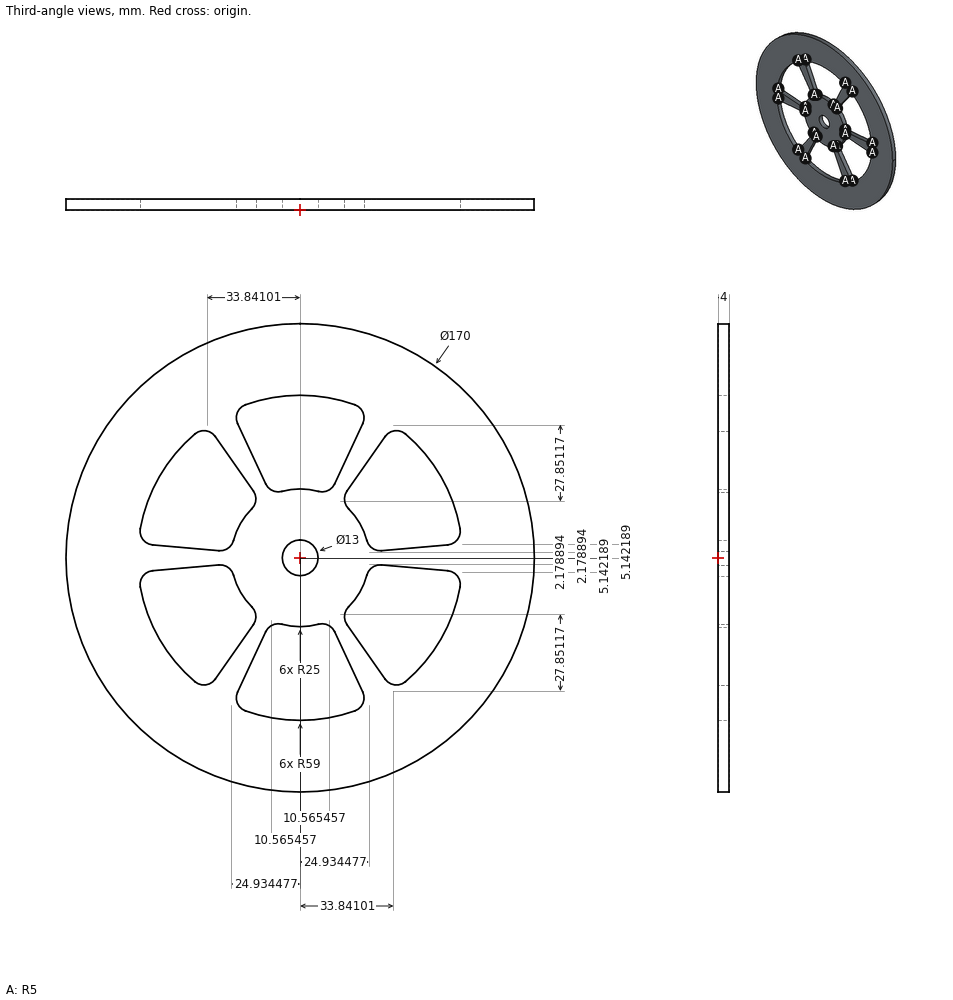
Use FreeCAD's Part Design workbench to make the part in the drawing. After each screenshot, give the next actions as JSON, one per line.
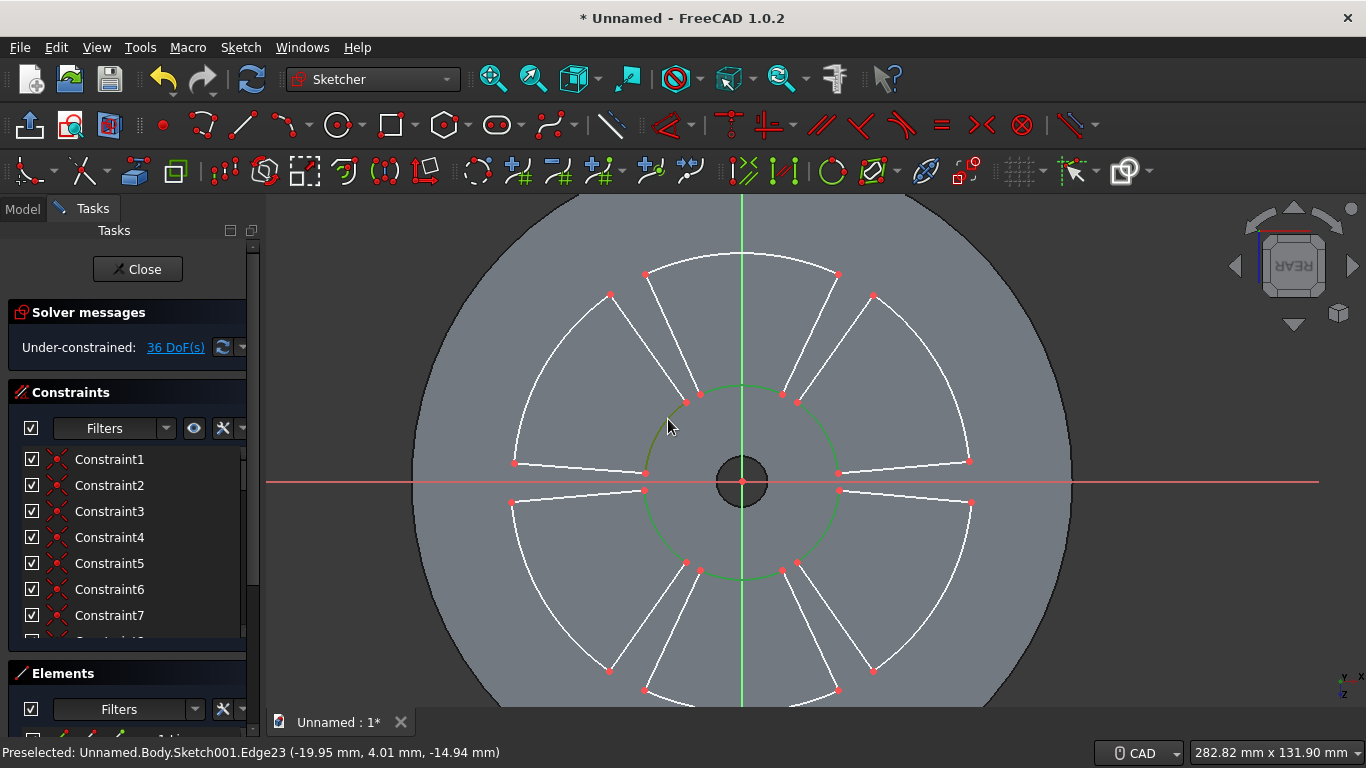
{"action": "left_click", "coordinate": [942, 126]}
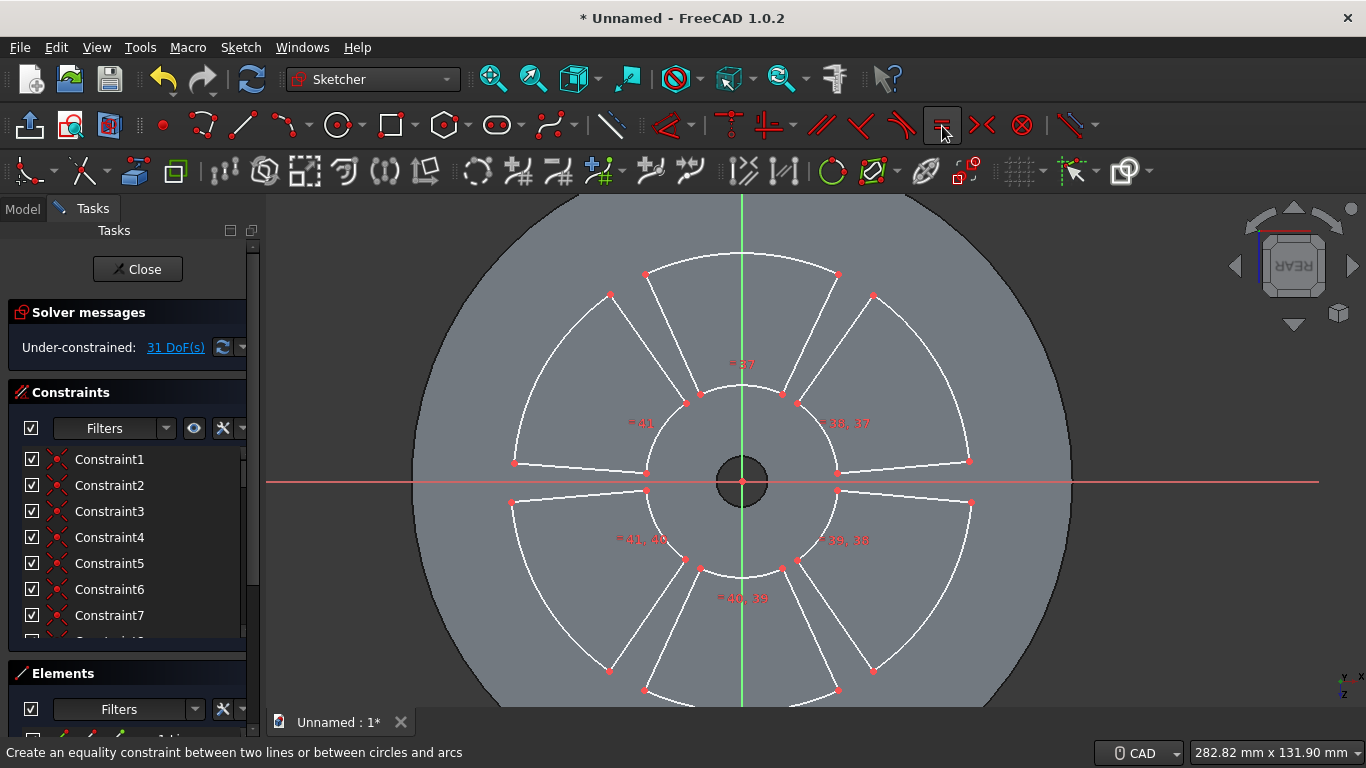
{"action": "left_click", "coordinate": [782, 257]}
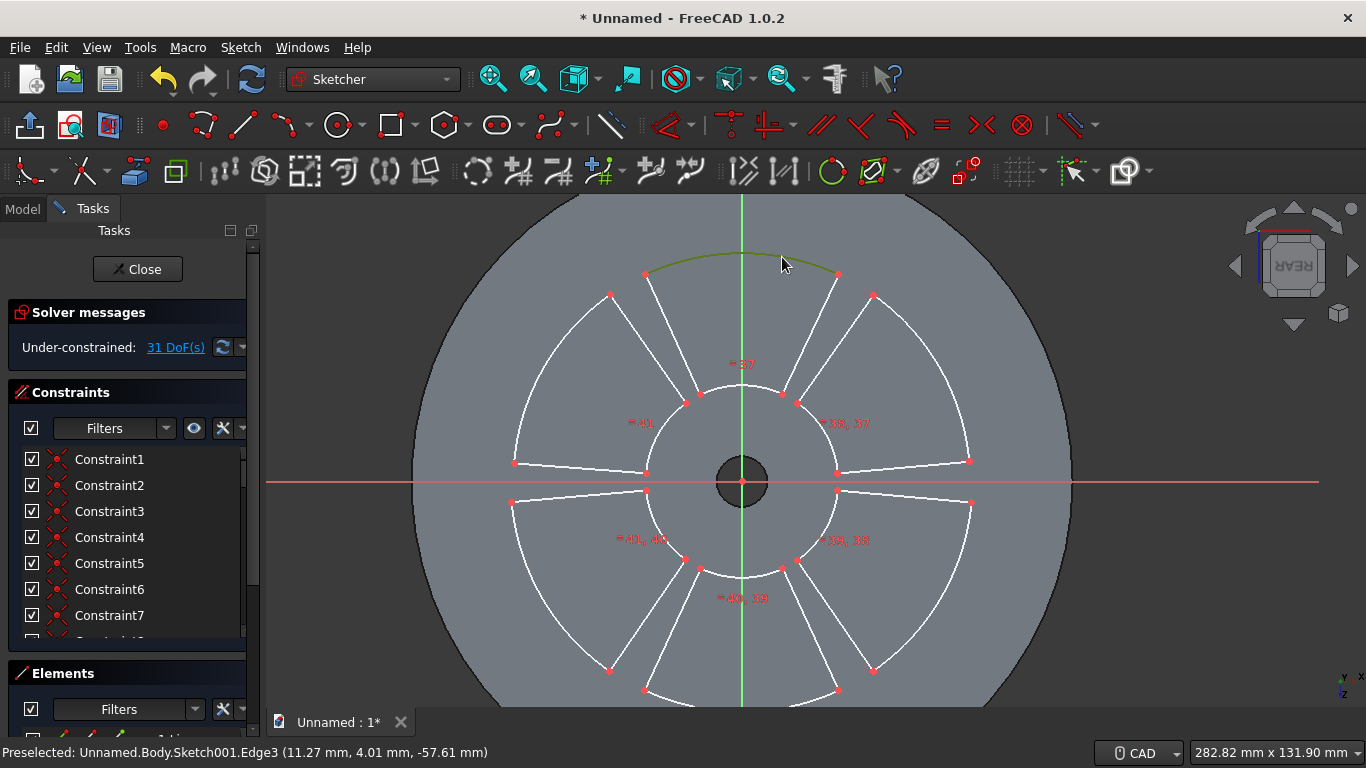
{"action": "left_click", "coordinate": [957, 404]}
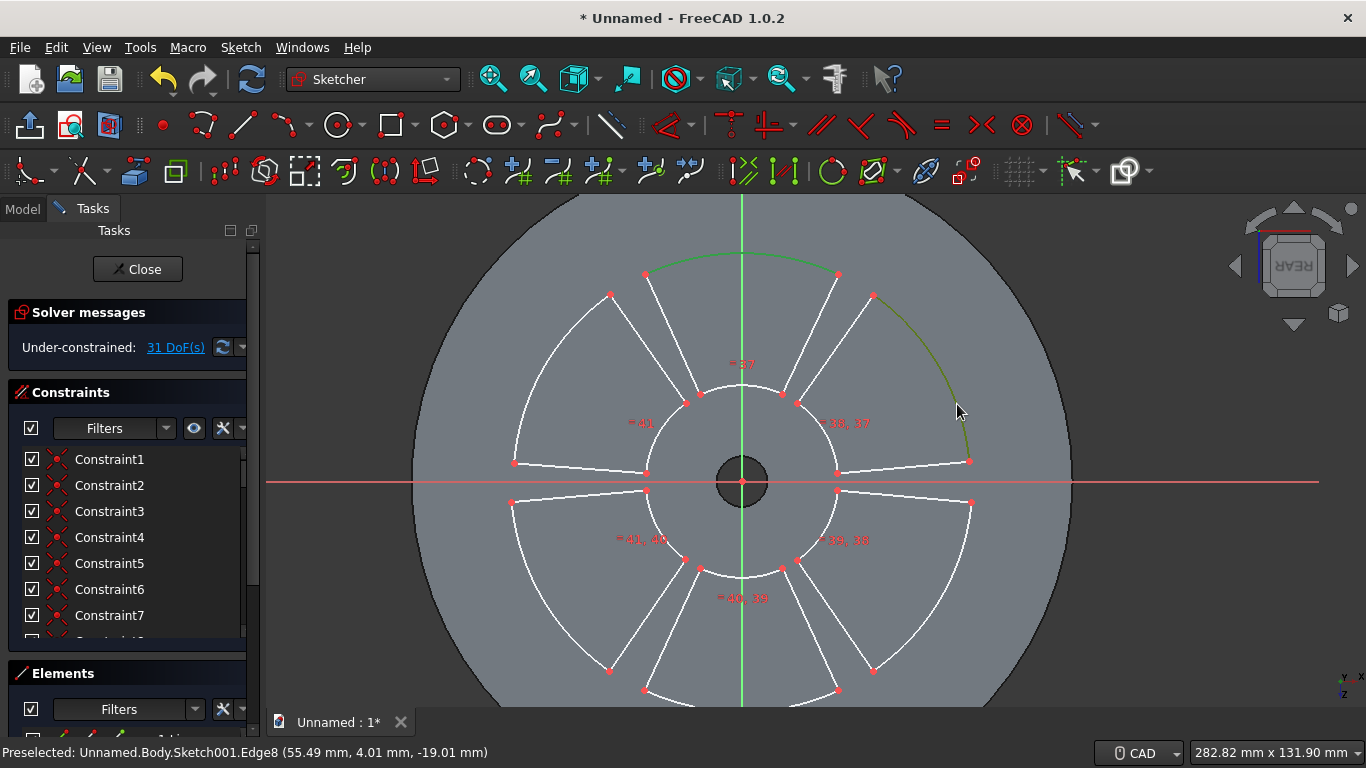
{"action": "left_click", "coordinate": [918, 631]}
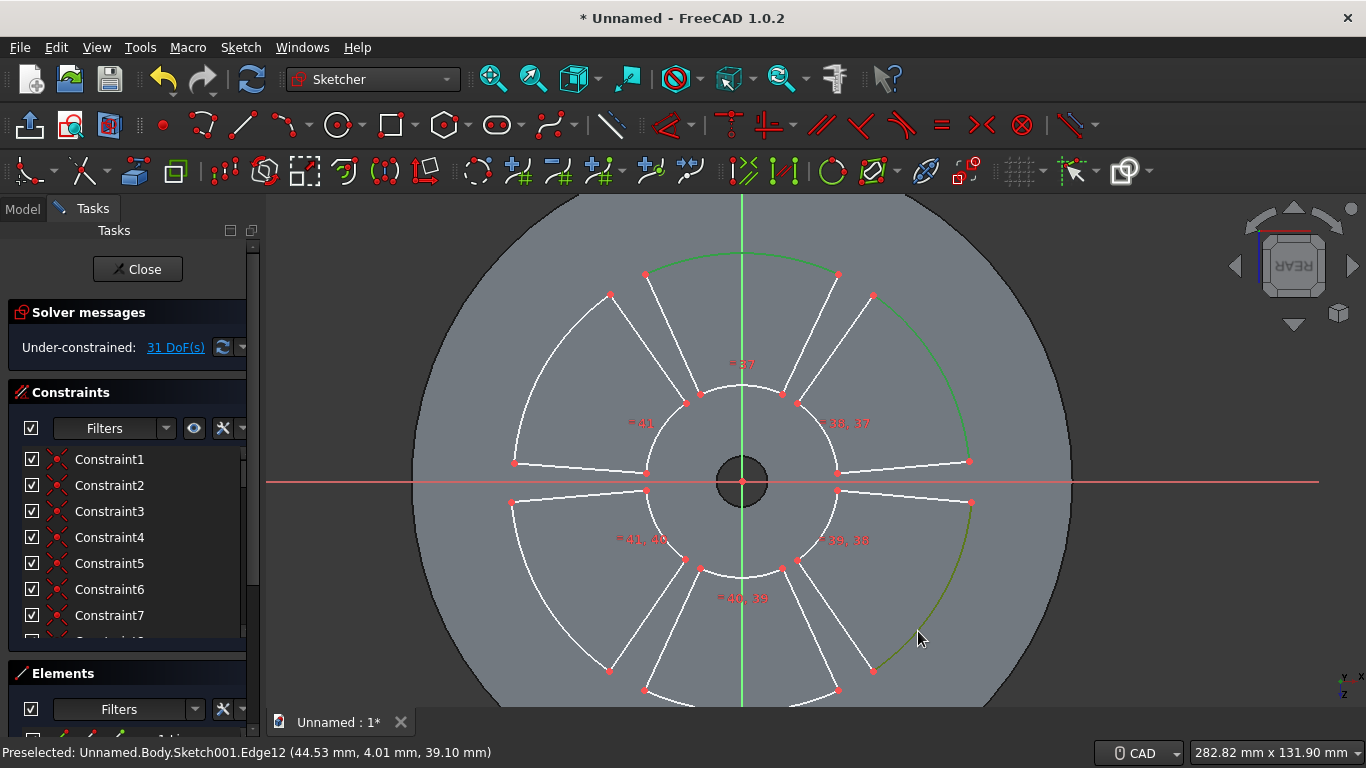
{"action": "scroll", "coordinate": [759, 387], "scroll_direction": "down", "scroll_amount": 2}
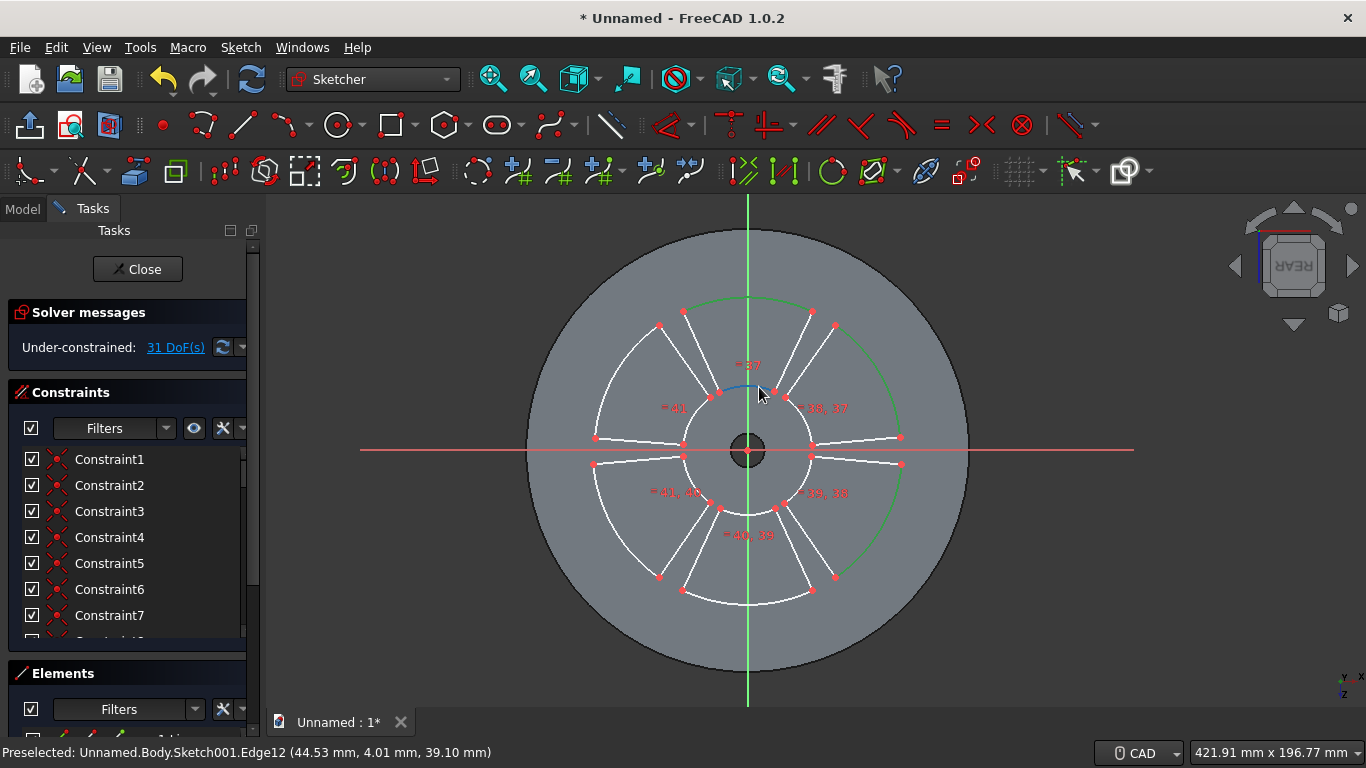
{"action": "left_click", "coordinate": [721, 602]}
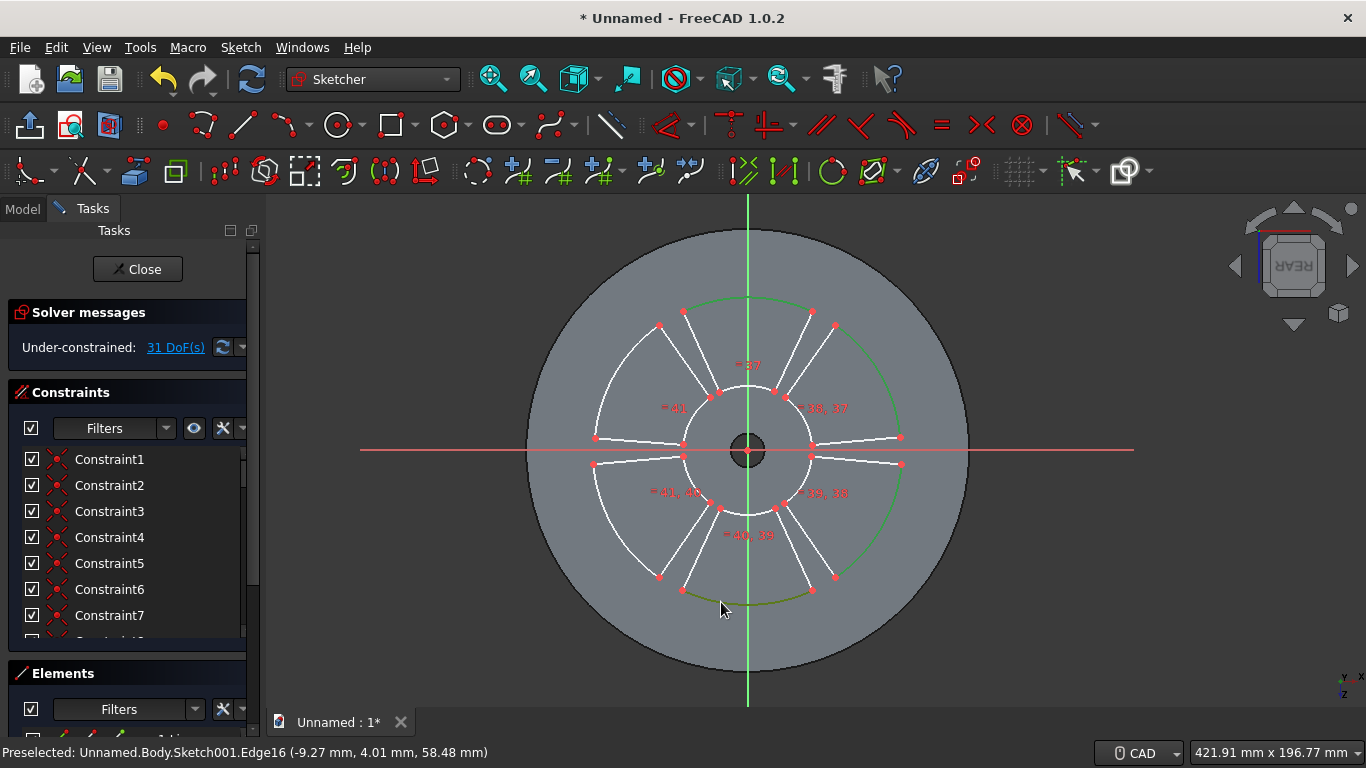
{"action": "left_click", "coordinate": [602, 504]}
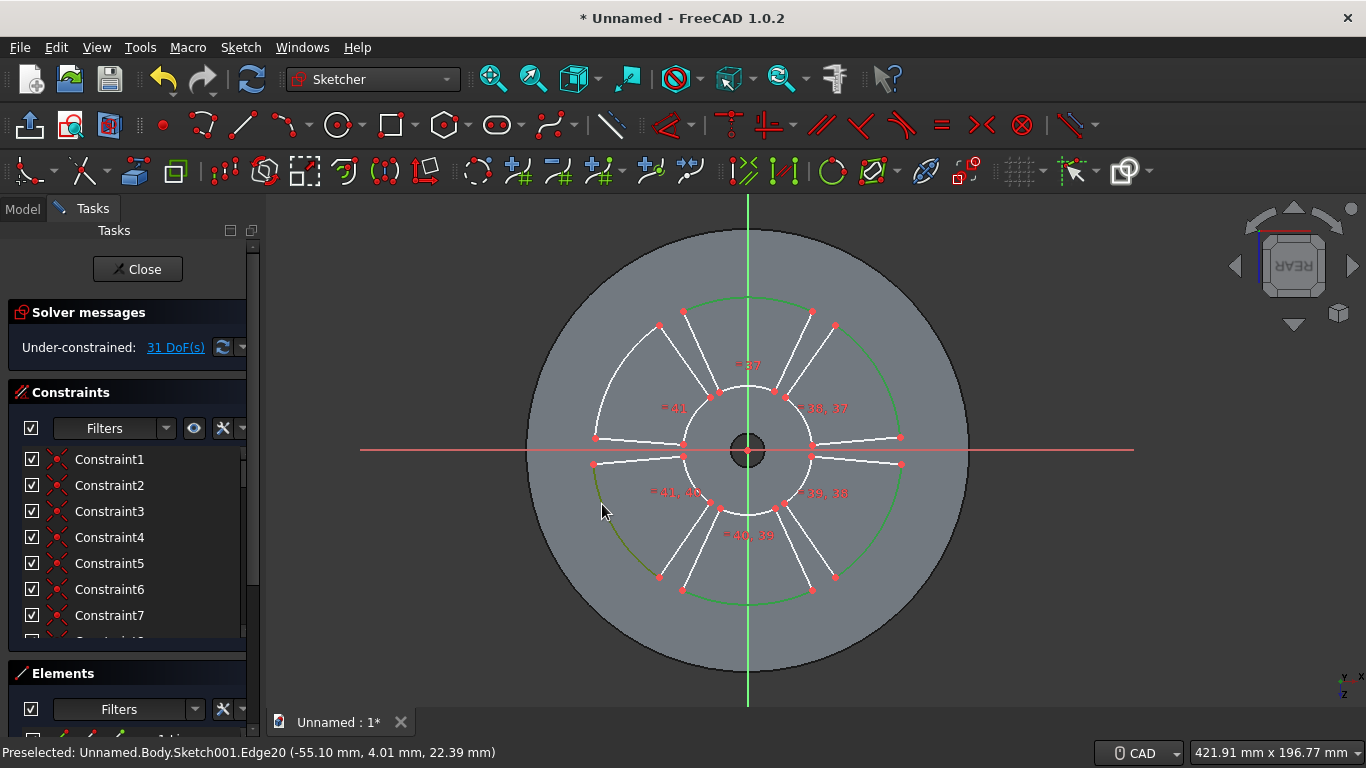
{"action": "left_click", "coordinate": [630, 353]}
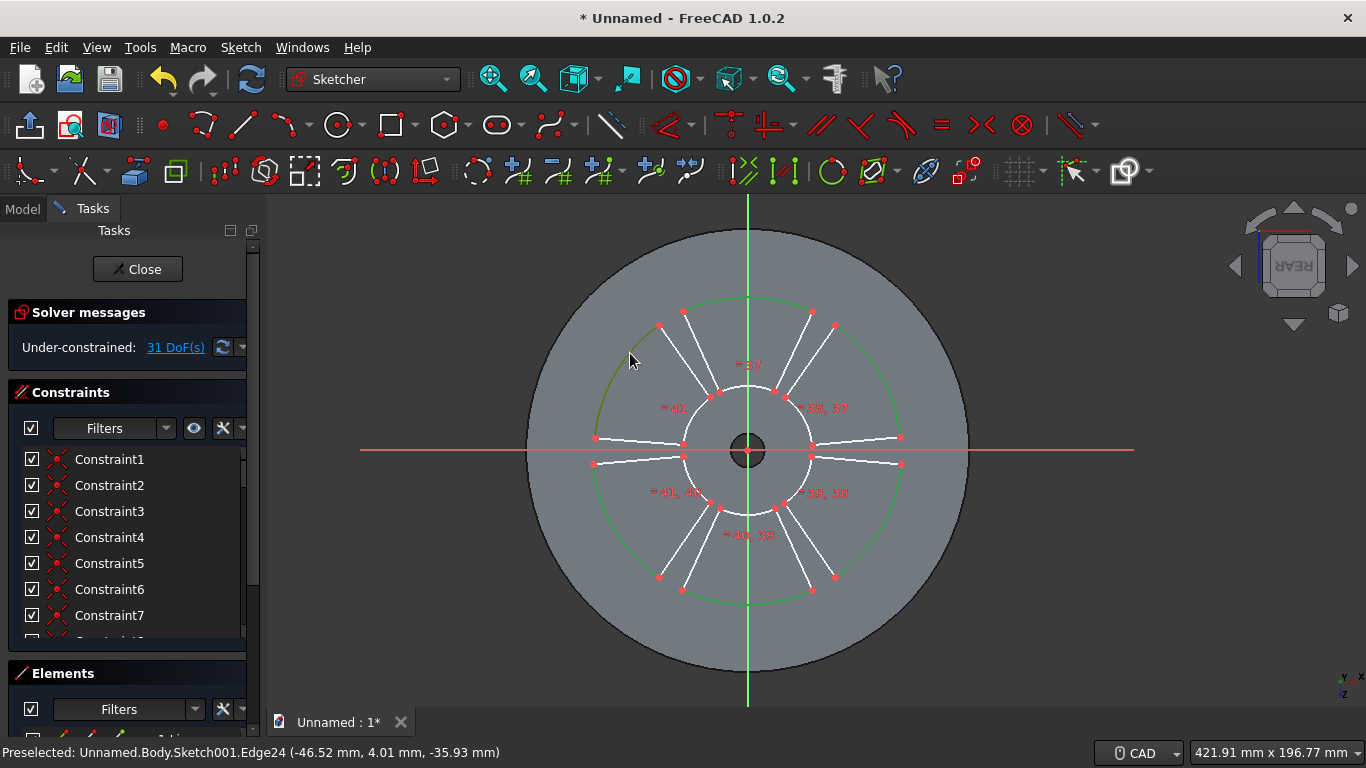
{"action": "left_click", "coordinate": [942, 126]}